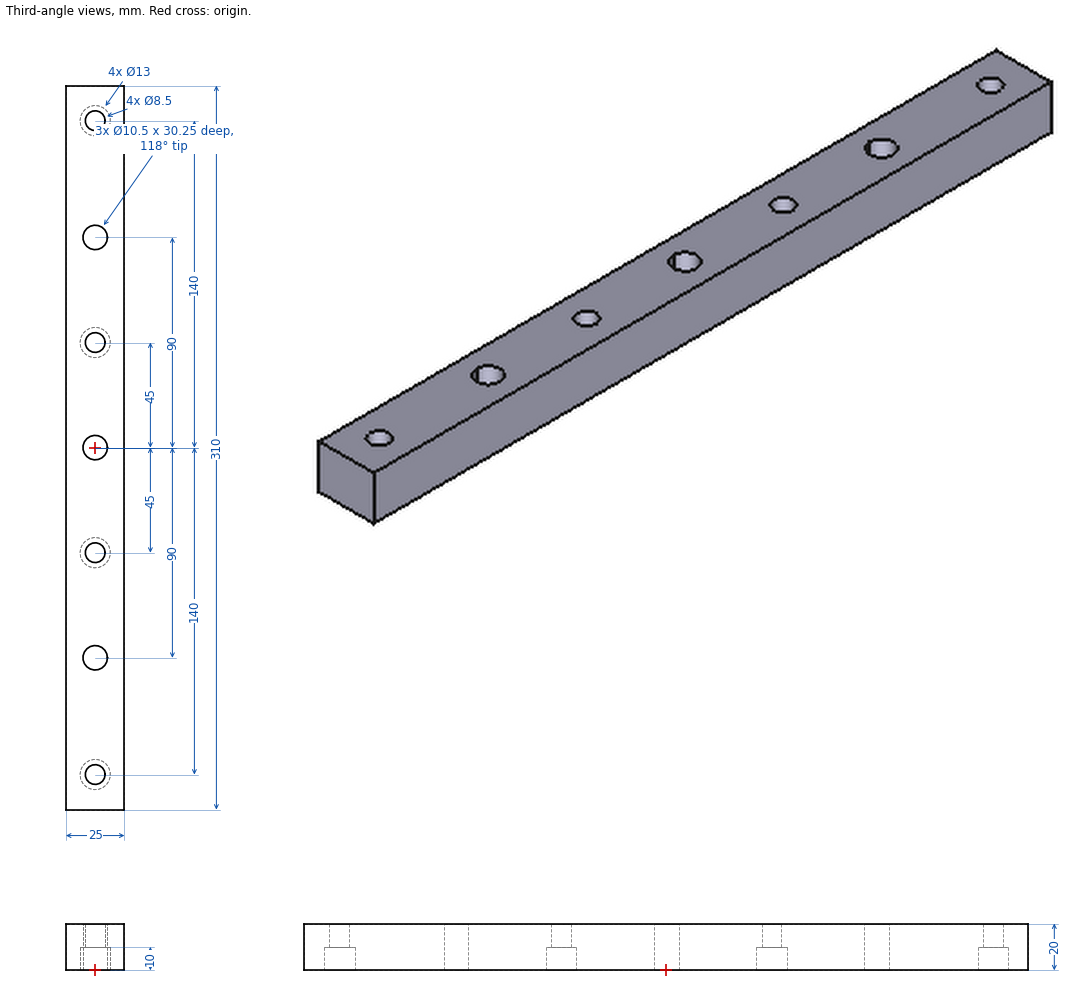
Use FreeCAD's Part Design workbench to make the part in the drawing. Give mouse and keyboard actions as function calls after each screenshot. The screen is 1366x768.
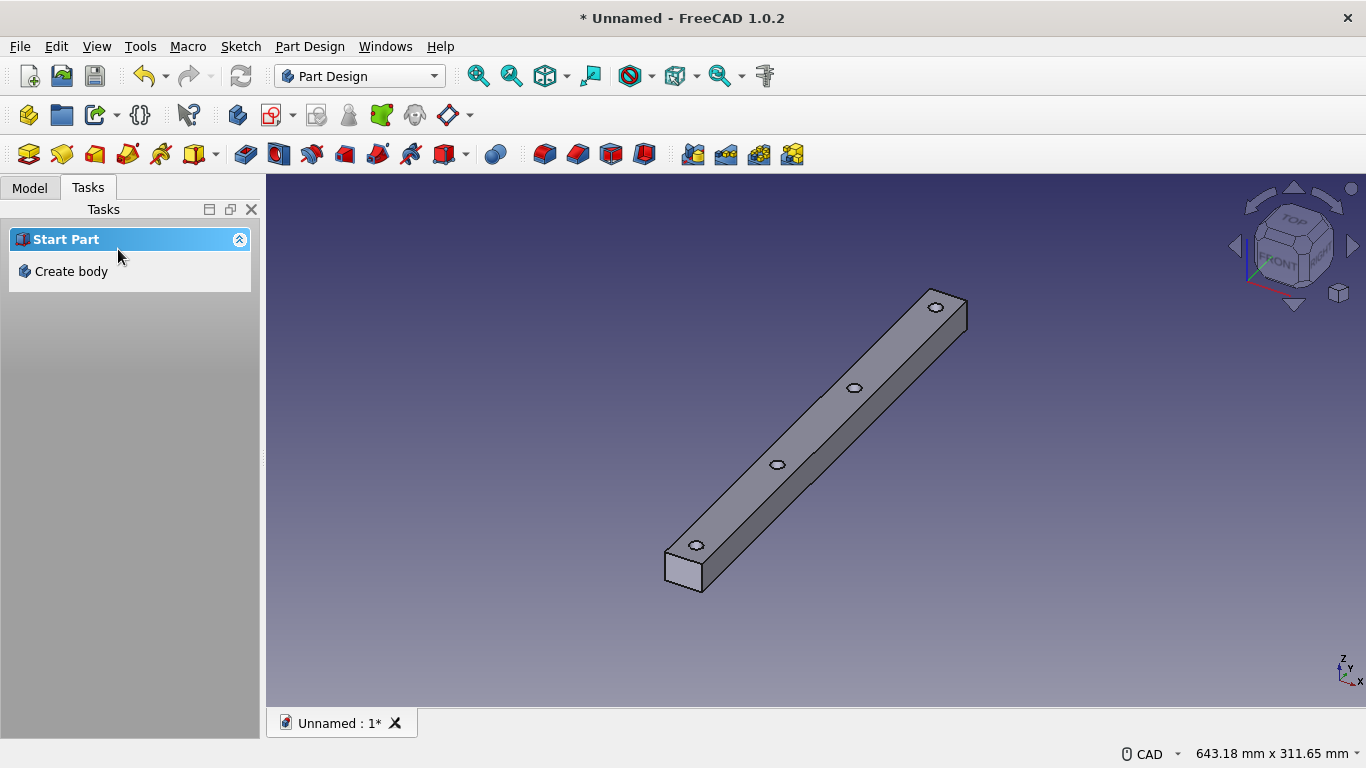
click(270, 116)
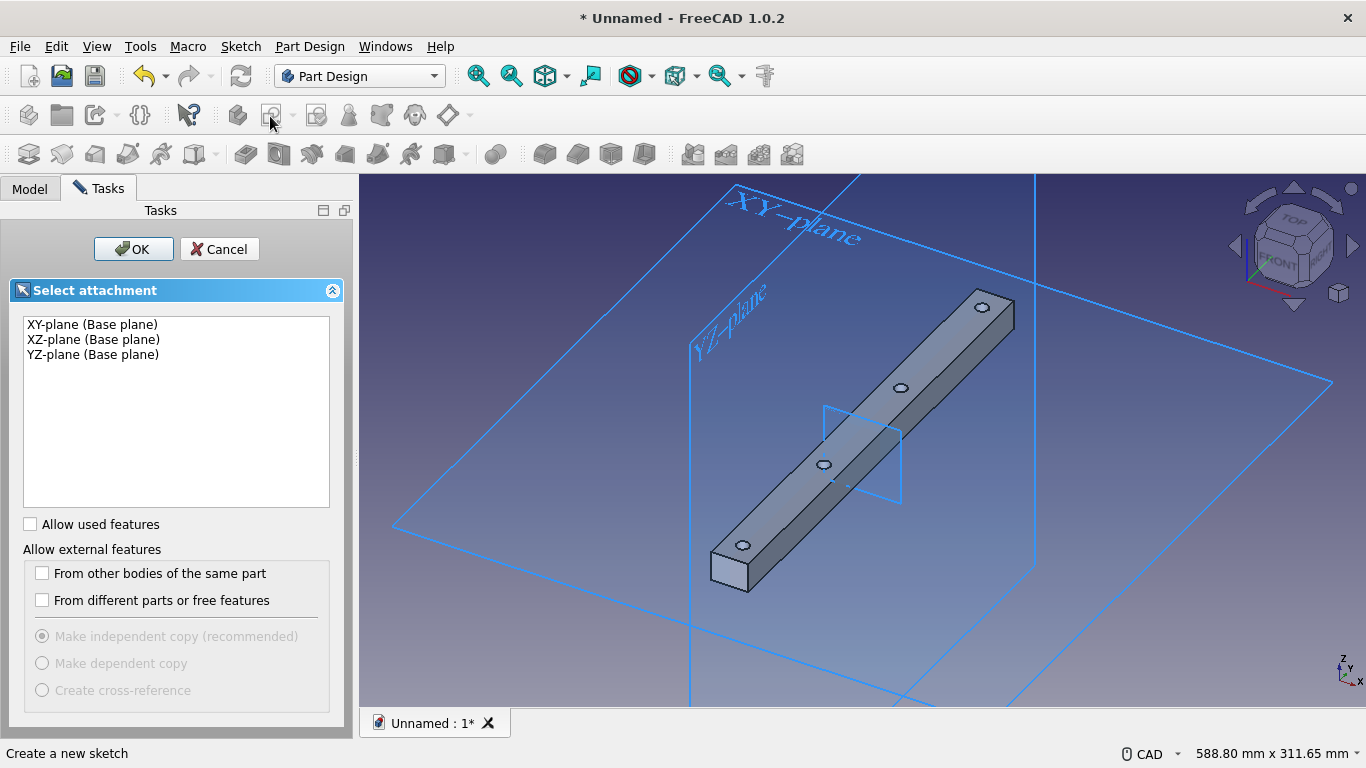
click(84, 324)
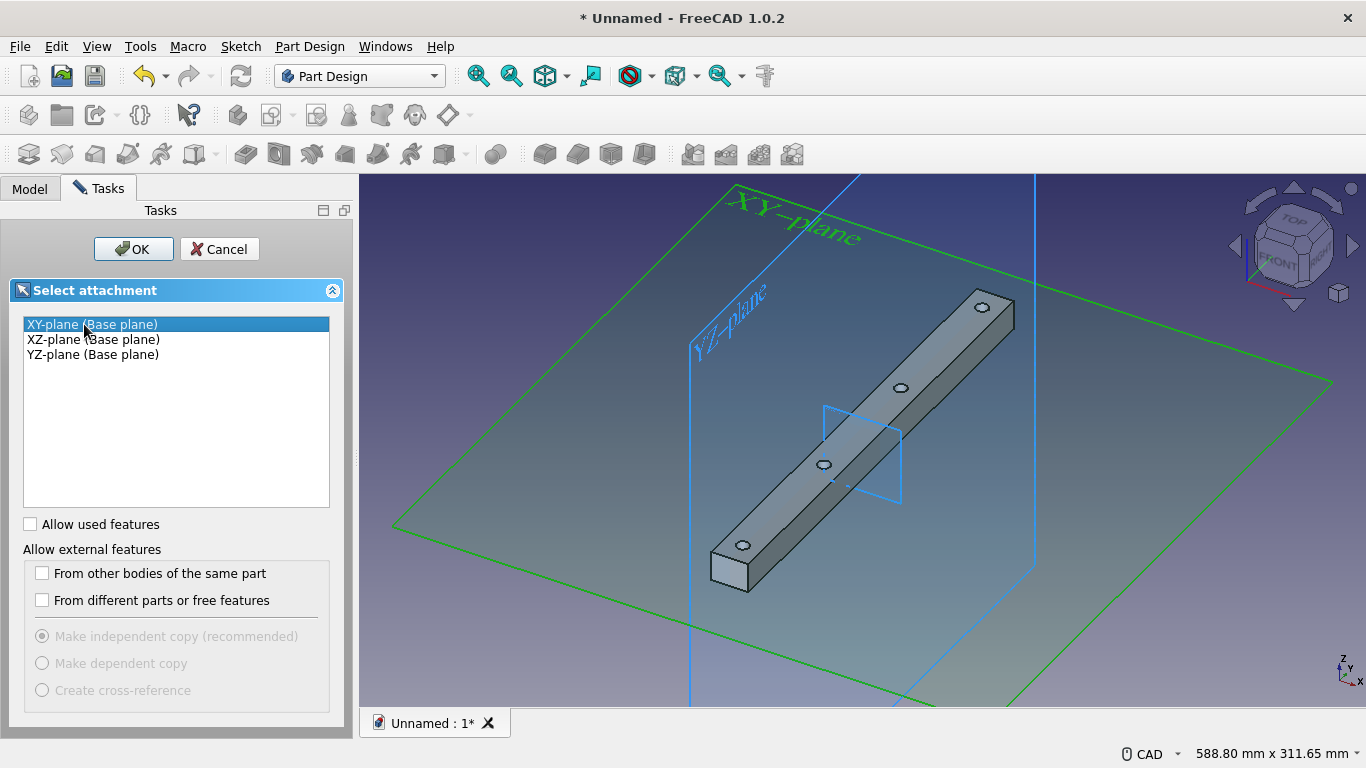
click(134, 249)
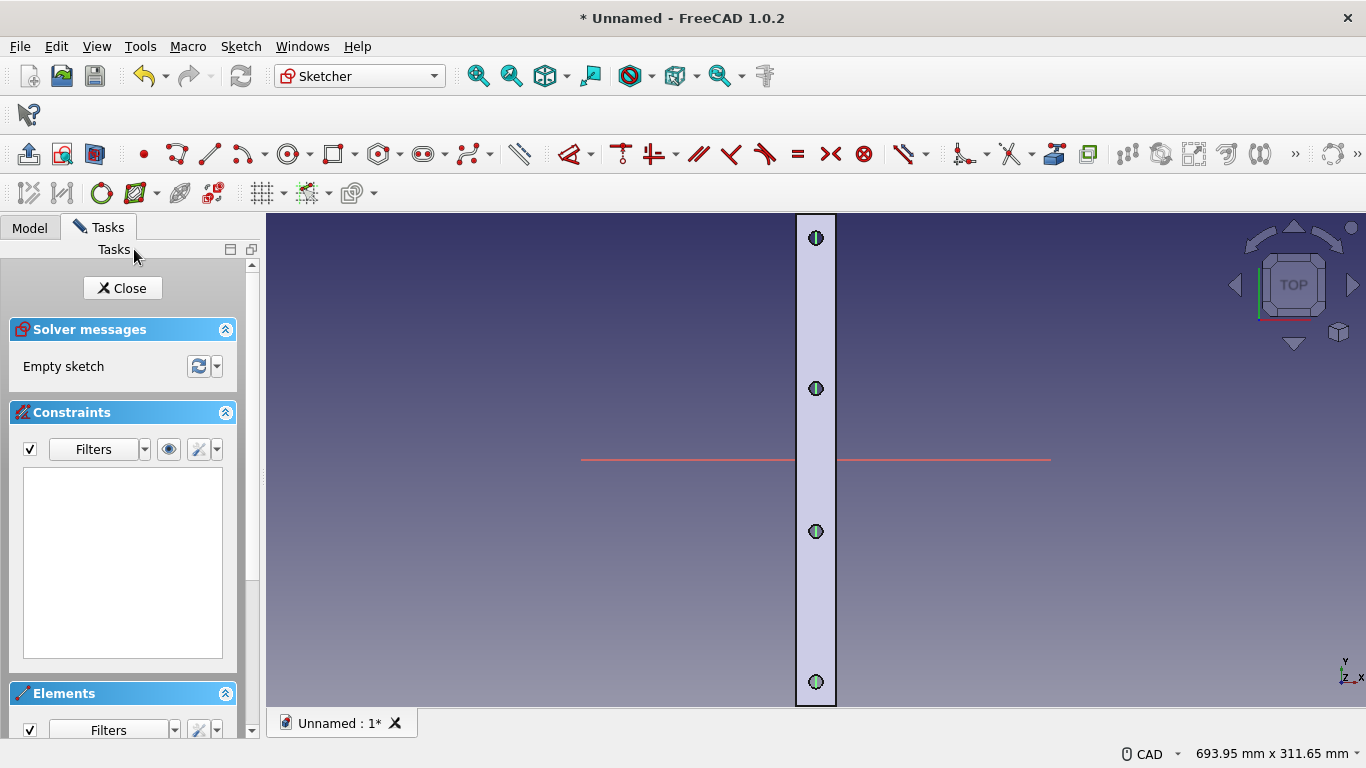
key(q)
key(s)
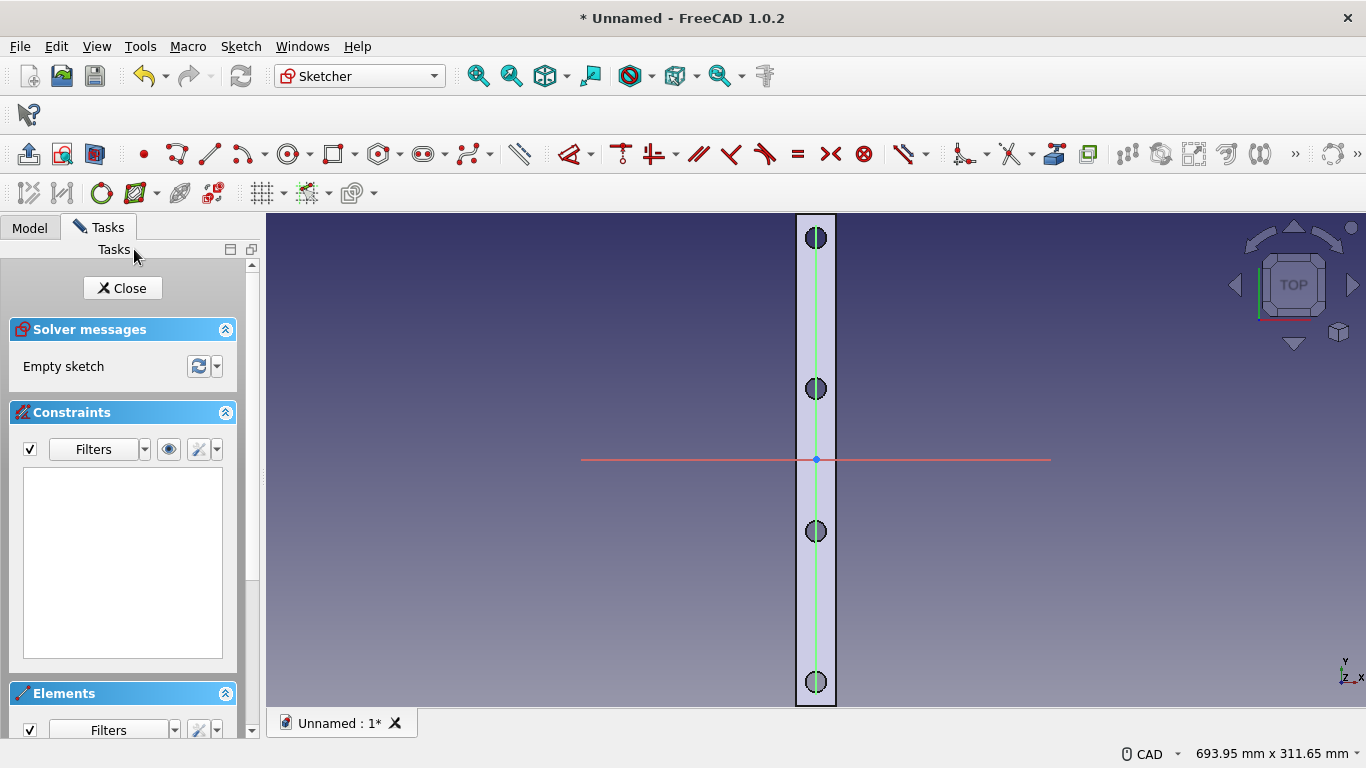
key(g)
key(c)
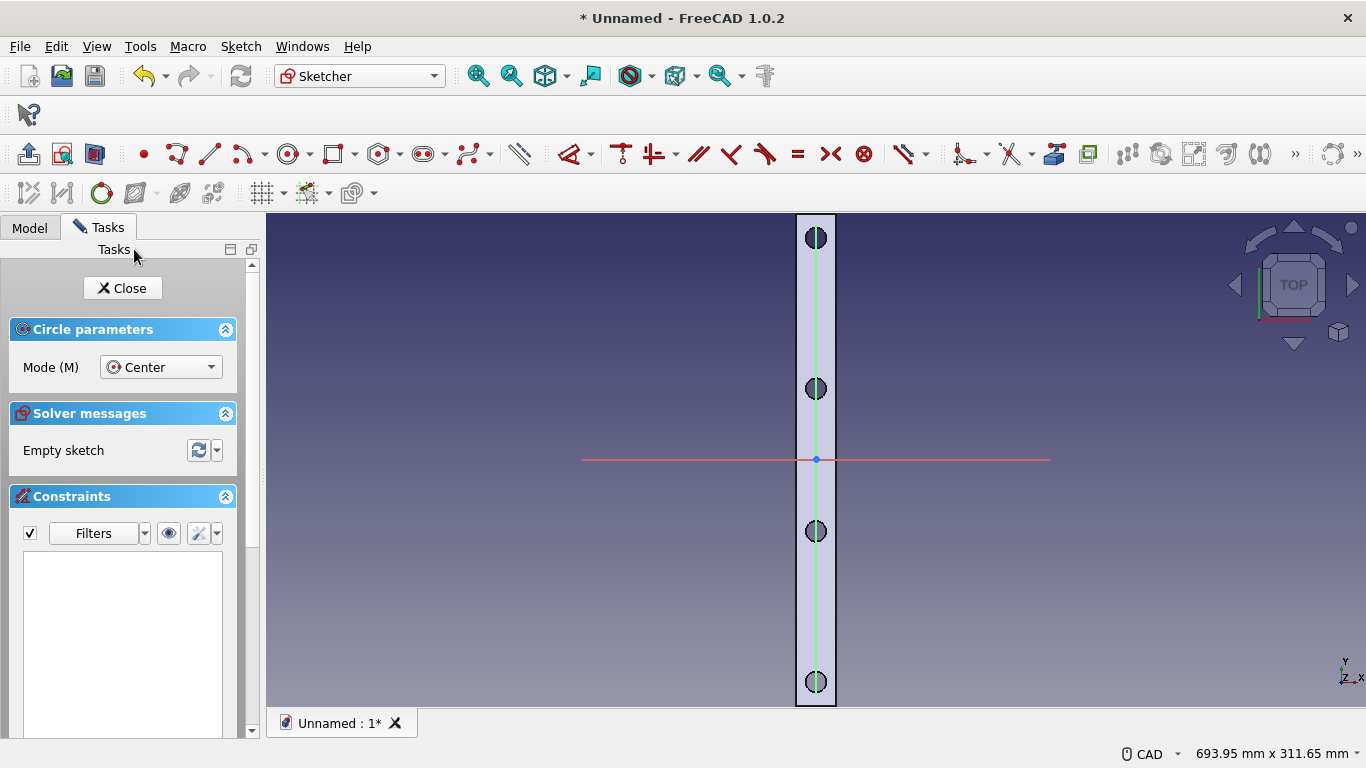
scroll(816, 317, up, 6)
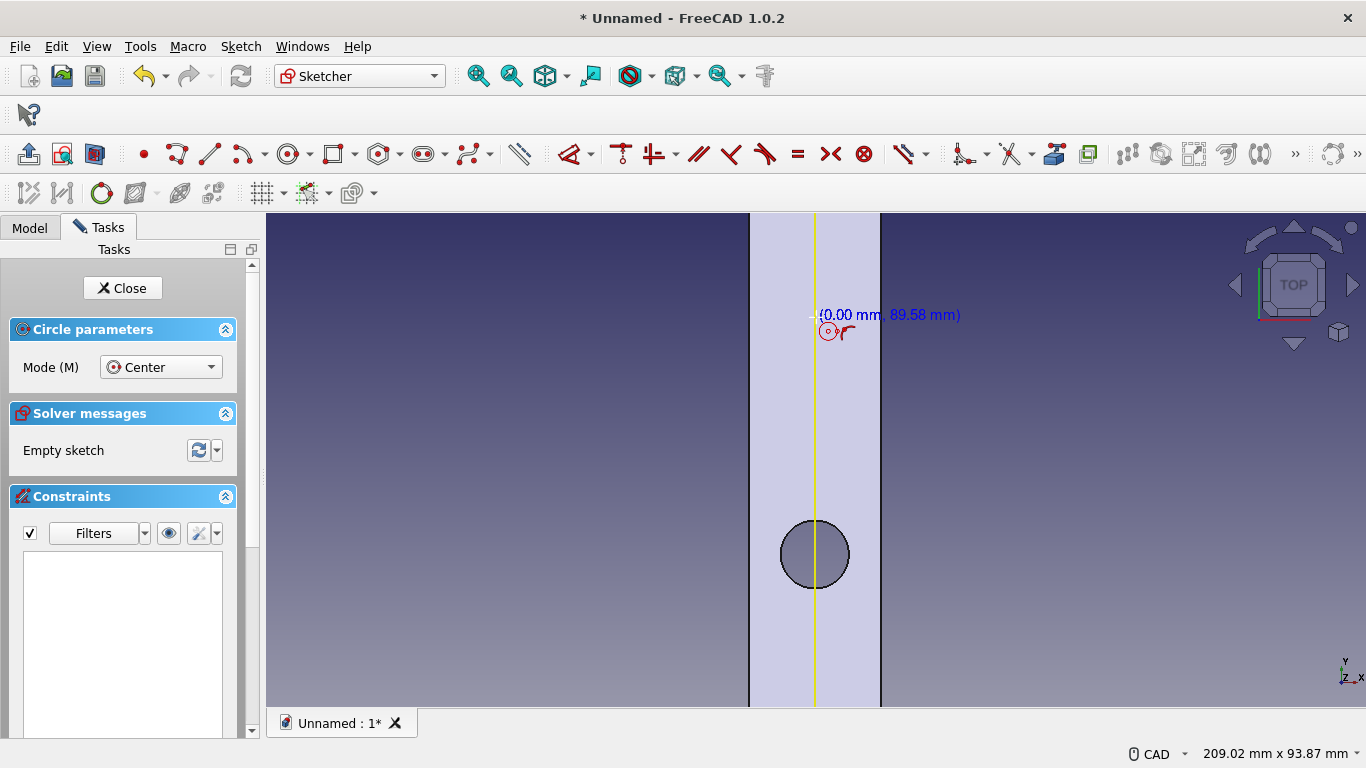
click(815, 318)
click(834, 298)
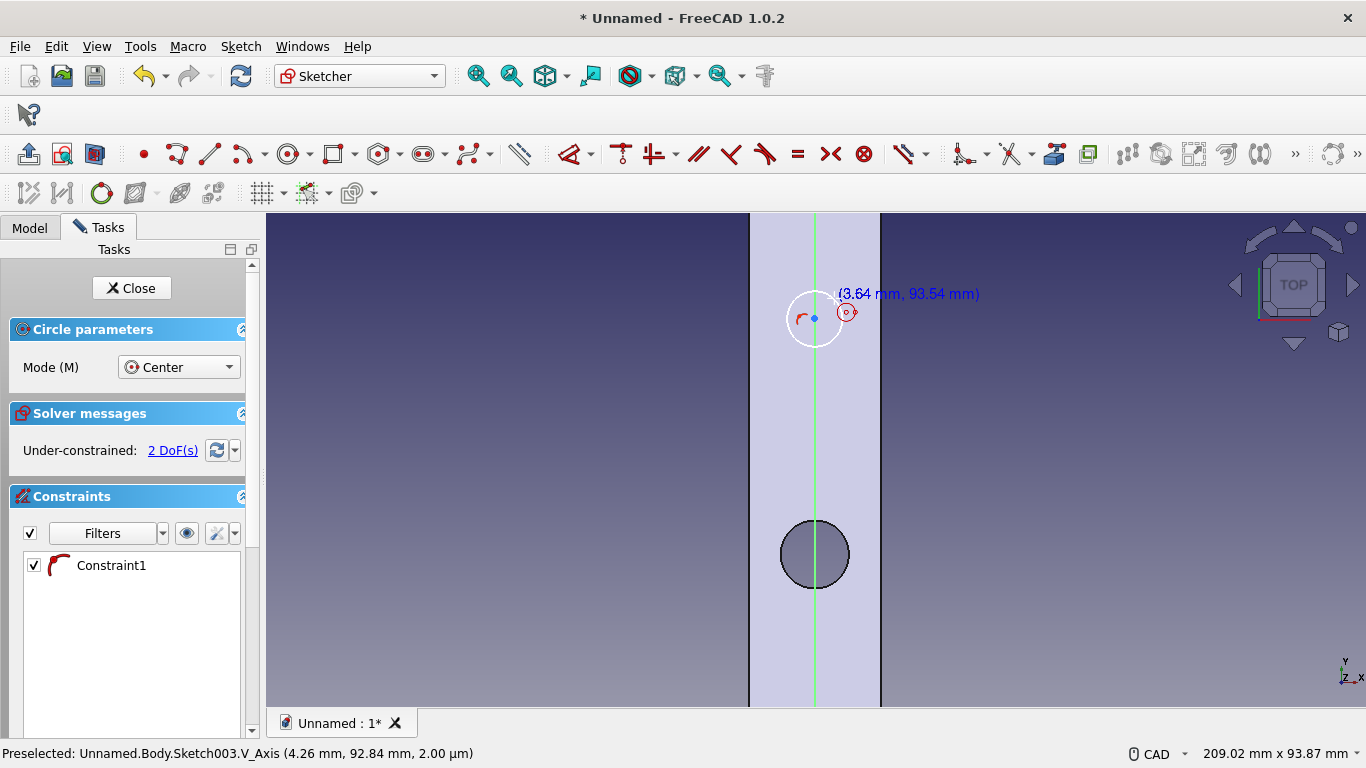
scroll(718, 317, down, 6)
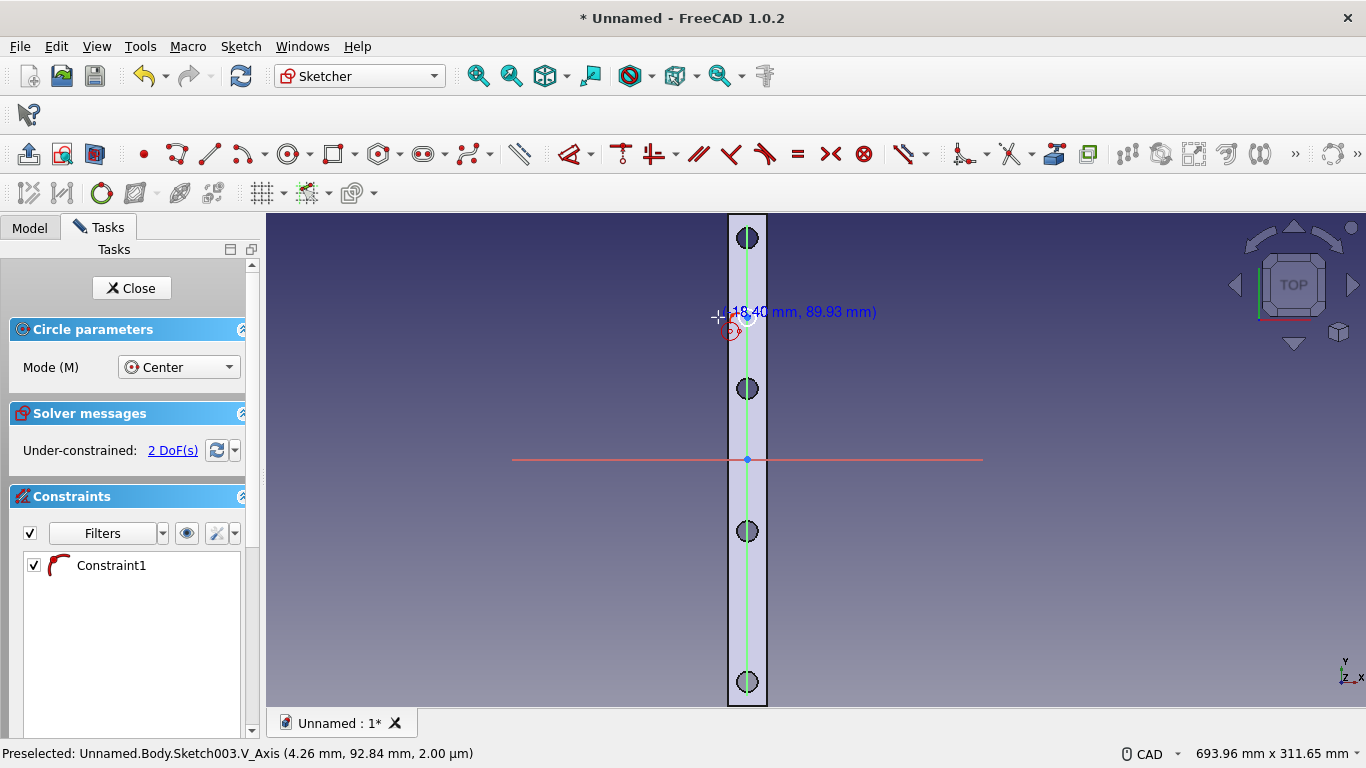
scroll(747, 460, up, 6)